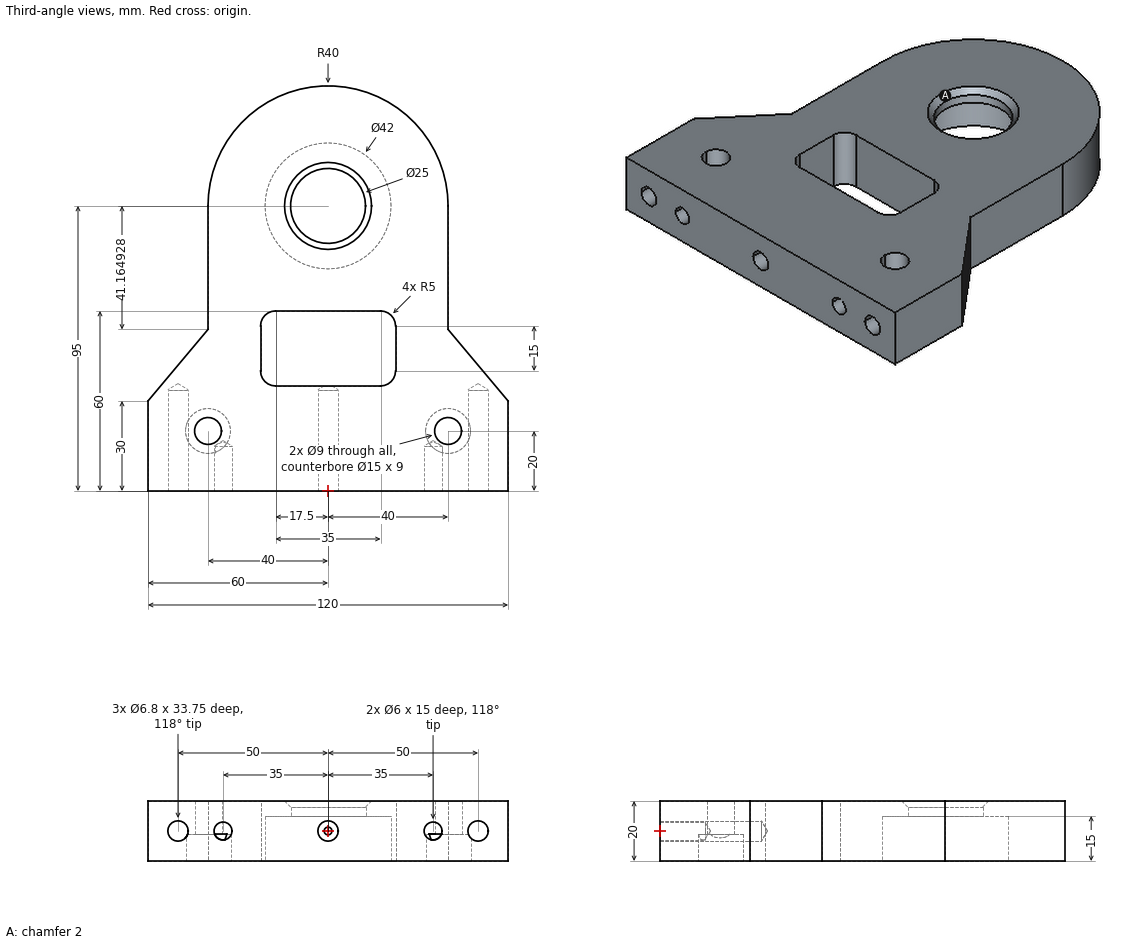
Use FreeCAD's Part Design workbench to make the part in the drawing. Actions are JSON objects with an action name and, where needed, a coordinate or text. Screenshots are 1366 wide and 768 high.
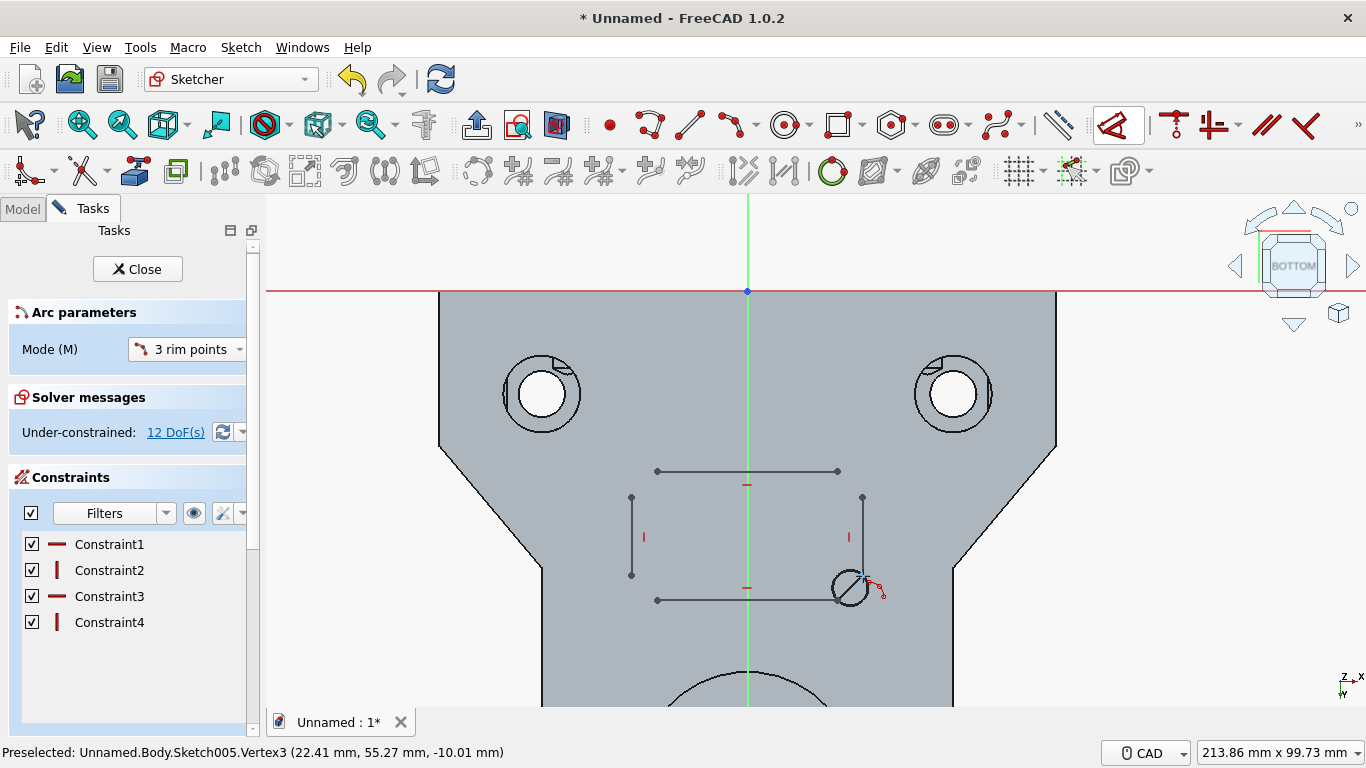
{"action": "scroll", "coordinate": [856, 592], "scroll_direction": "up", "scroll_amount": 4}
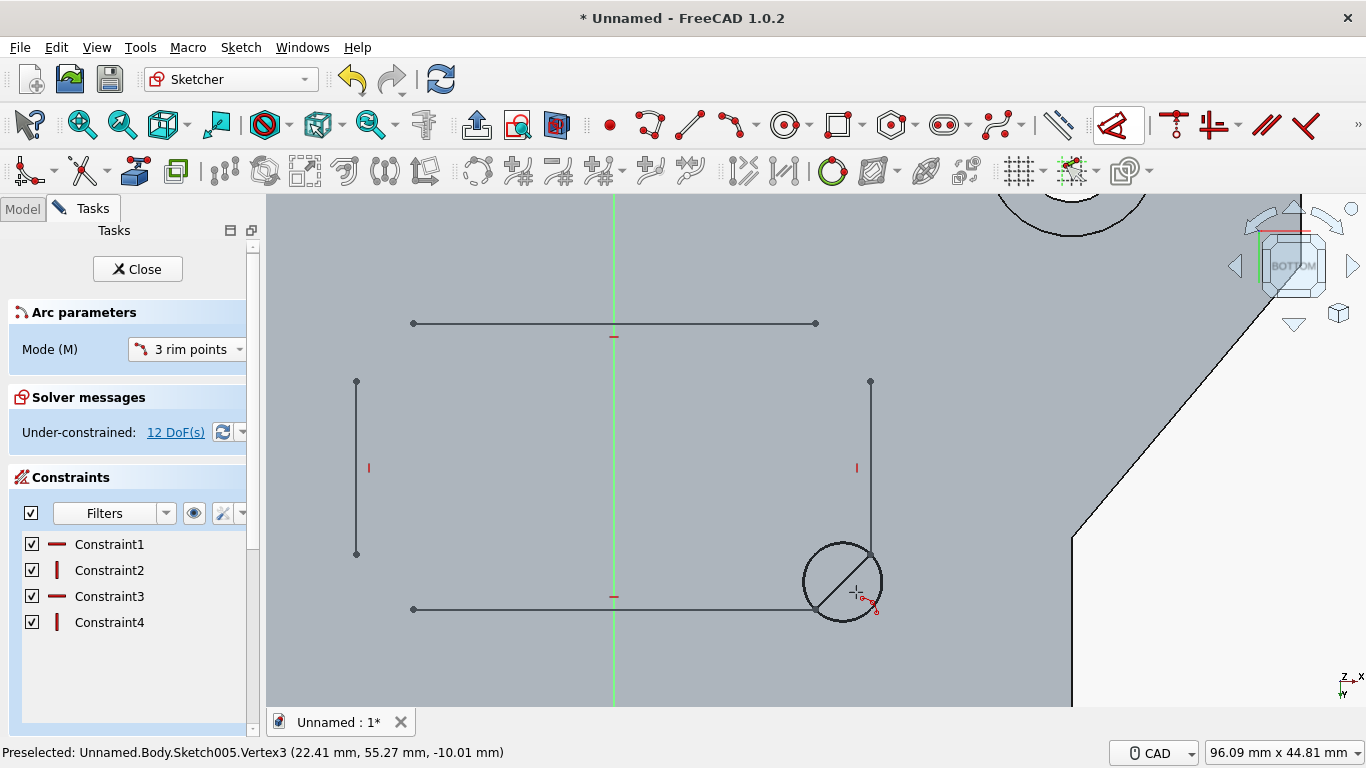
{"action": "left_click", "coordinate": [855, 592]}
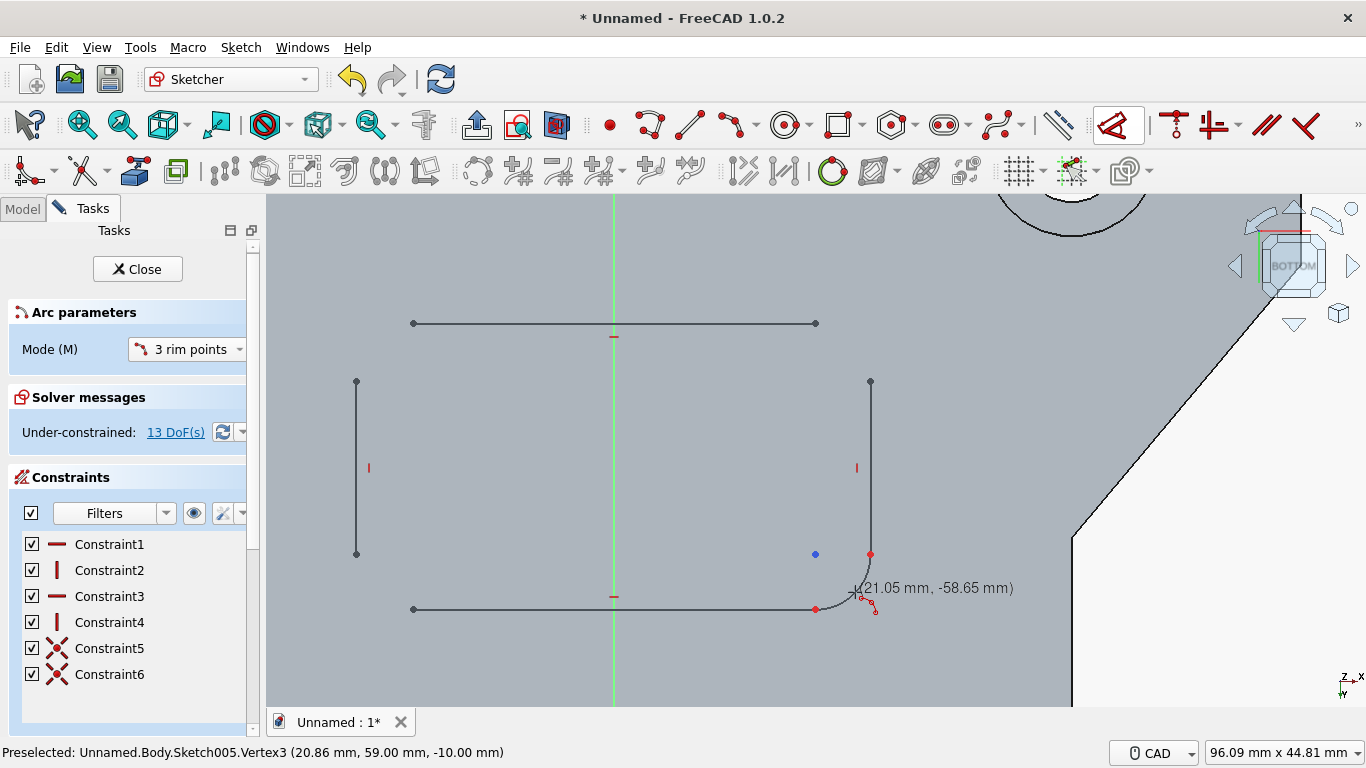
{"action": "left_click", "coordinate": [871, 381]}
{"action": "left_click", "coordinate": [815, 324]}
{"action": "left_click", "coordinate": [855, 339]}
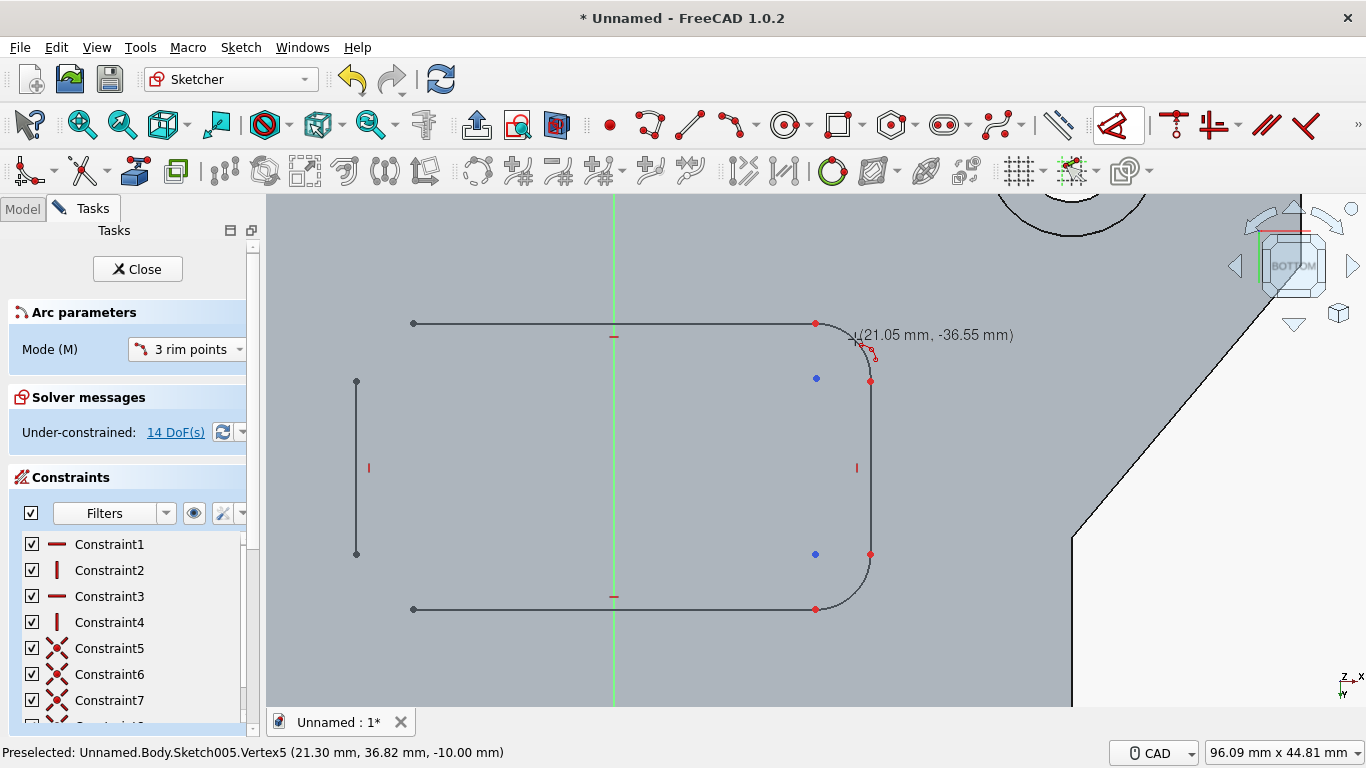
{"action": "left_click", "coordinate": [414, 324]}
{"action": "left_click", "coordinate": [356, 381]}
{"action": "left_click", "coordinate": [373, 339]}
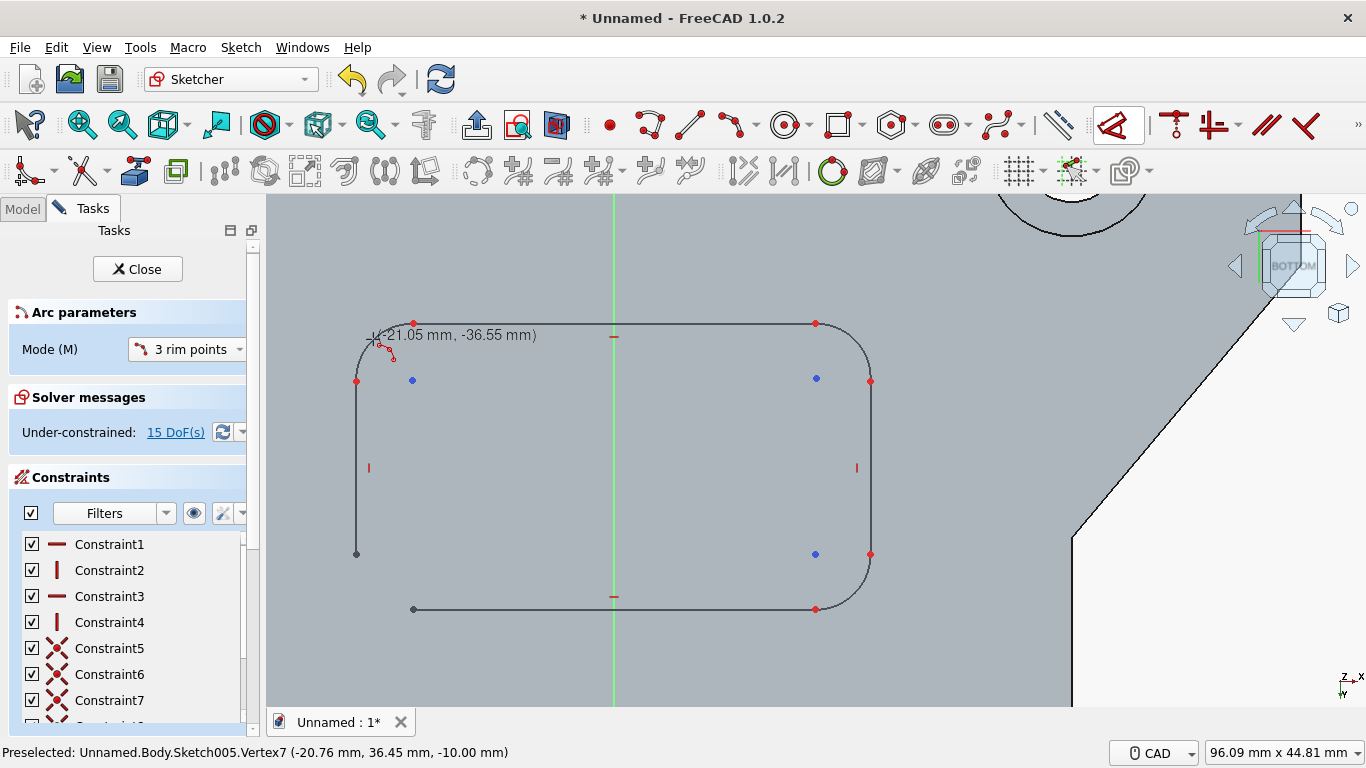
{"action": "left_click", "coordinate": [356, 554]}
{"action": "left_click", "coordinate": [414, 610]}
{"action": "left_click", "coordinate": [373, 592]}
{"action": "key", "text": "Escape"}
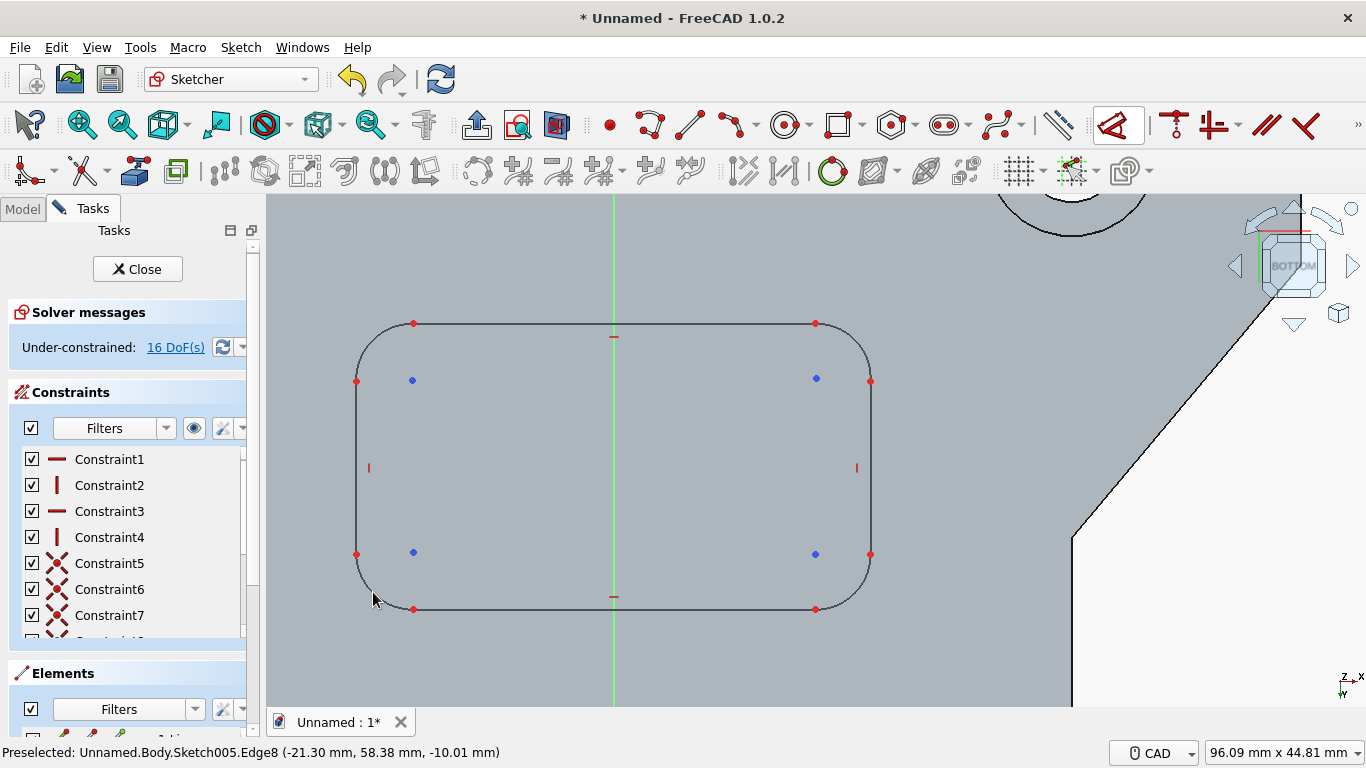
{"action": "left_click", "coordinate": [534, 610]}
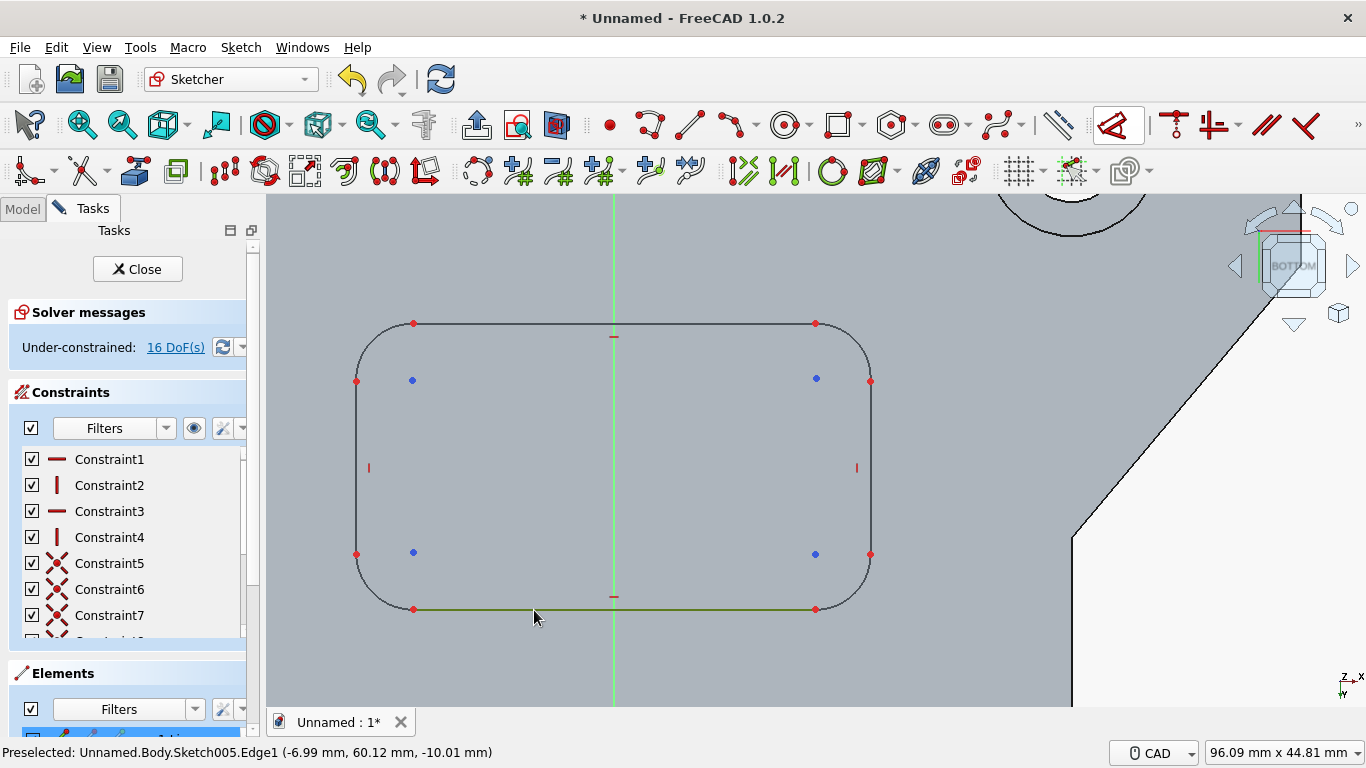
{"action": "left_click", "coordinate": [840, 604]}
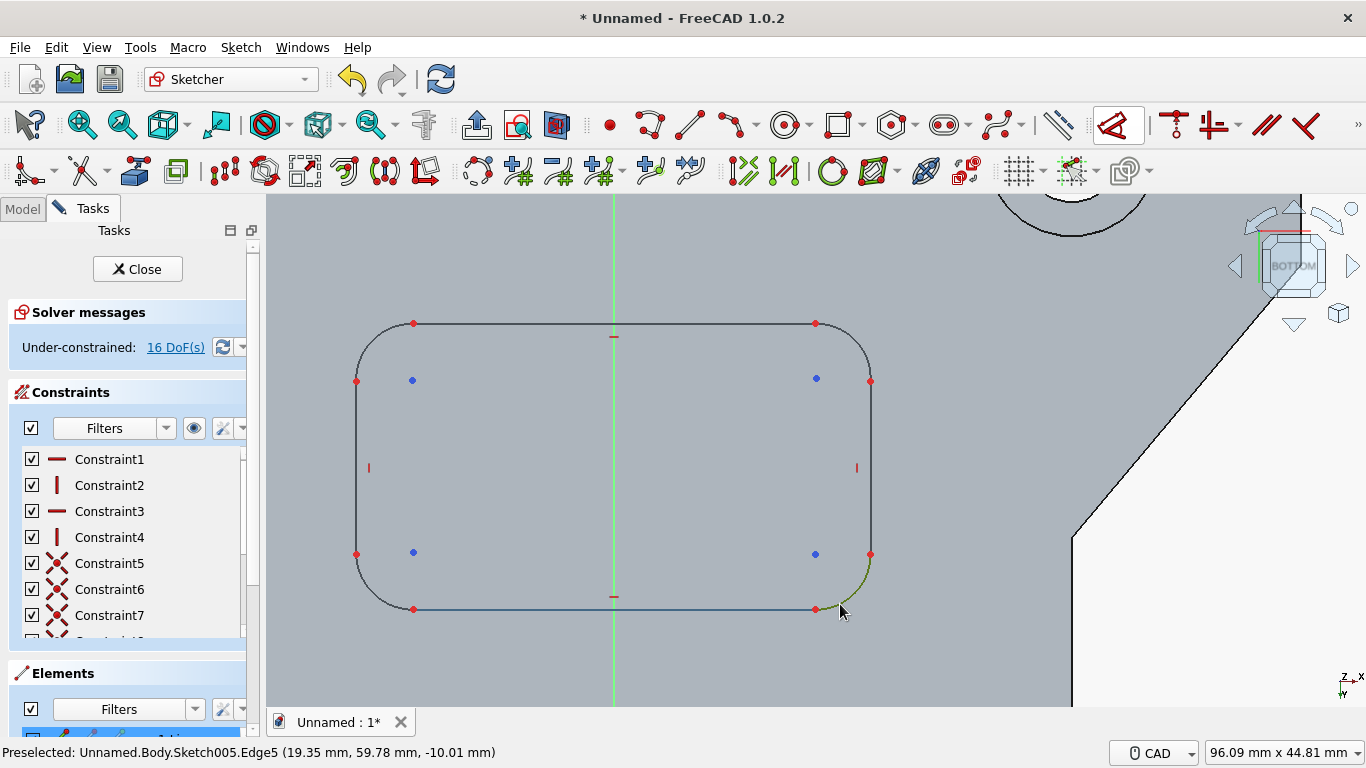
{"action": "key", "text": "t"}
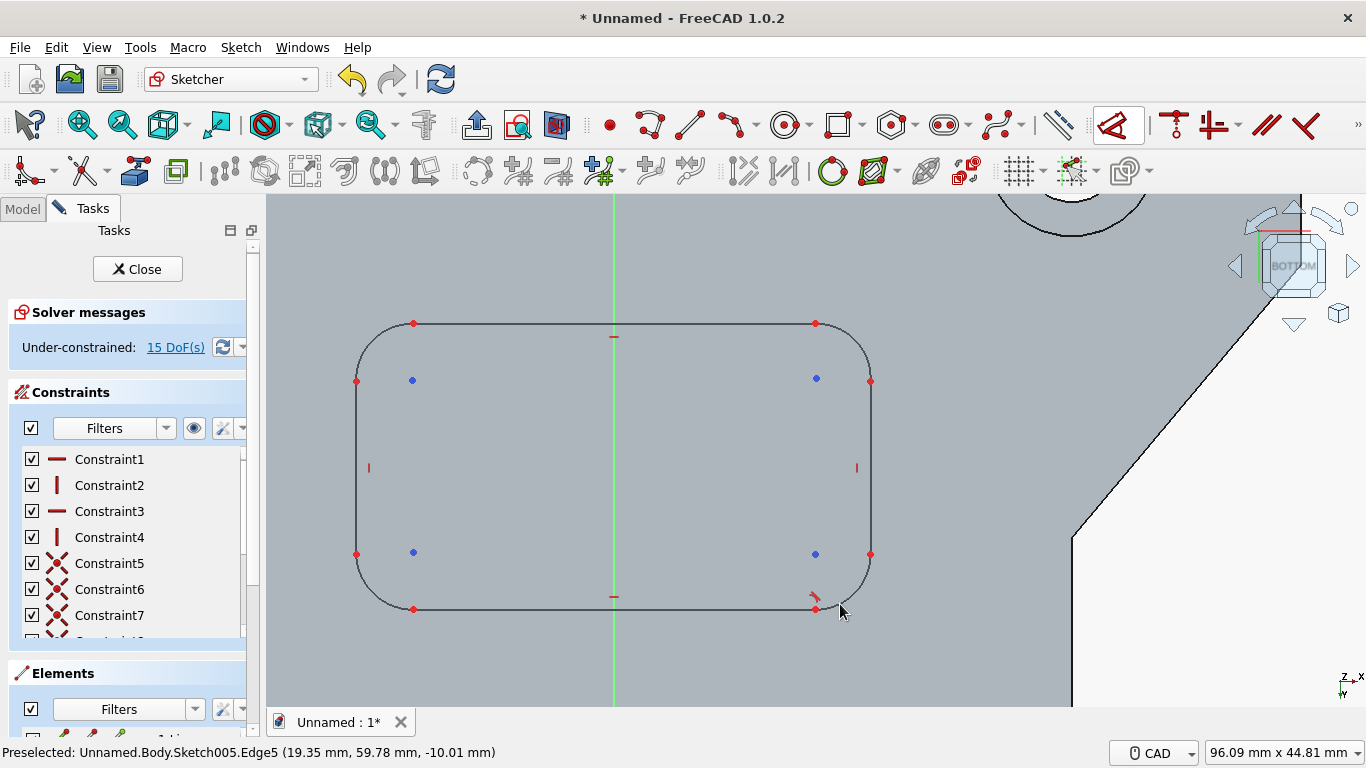
{"action": "left_click", "coordinate": [534, 610]}